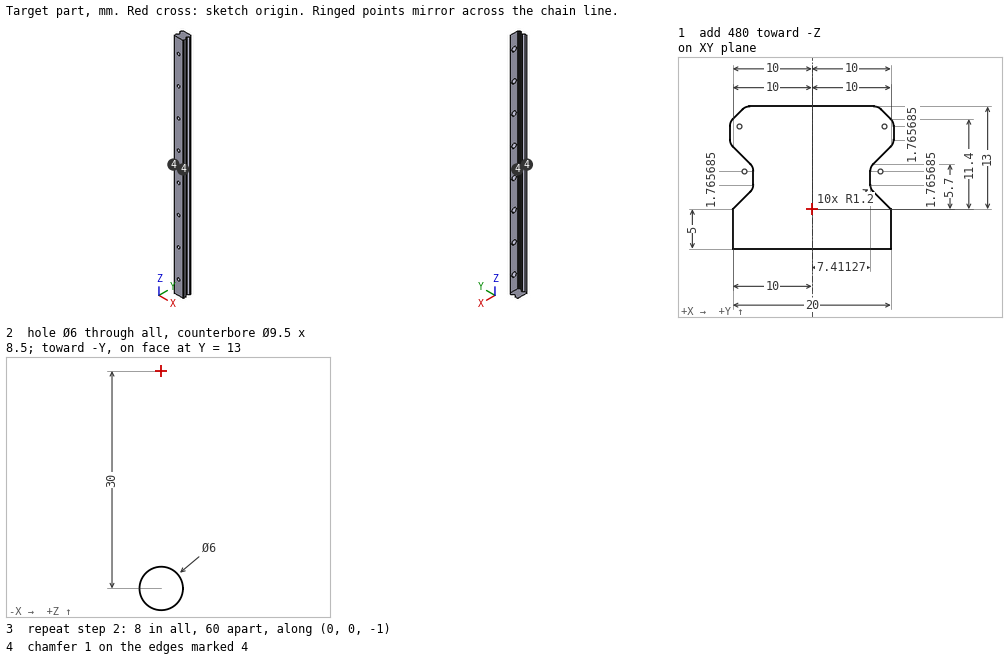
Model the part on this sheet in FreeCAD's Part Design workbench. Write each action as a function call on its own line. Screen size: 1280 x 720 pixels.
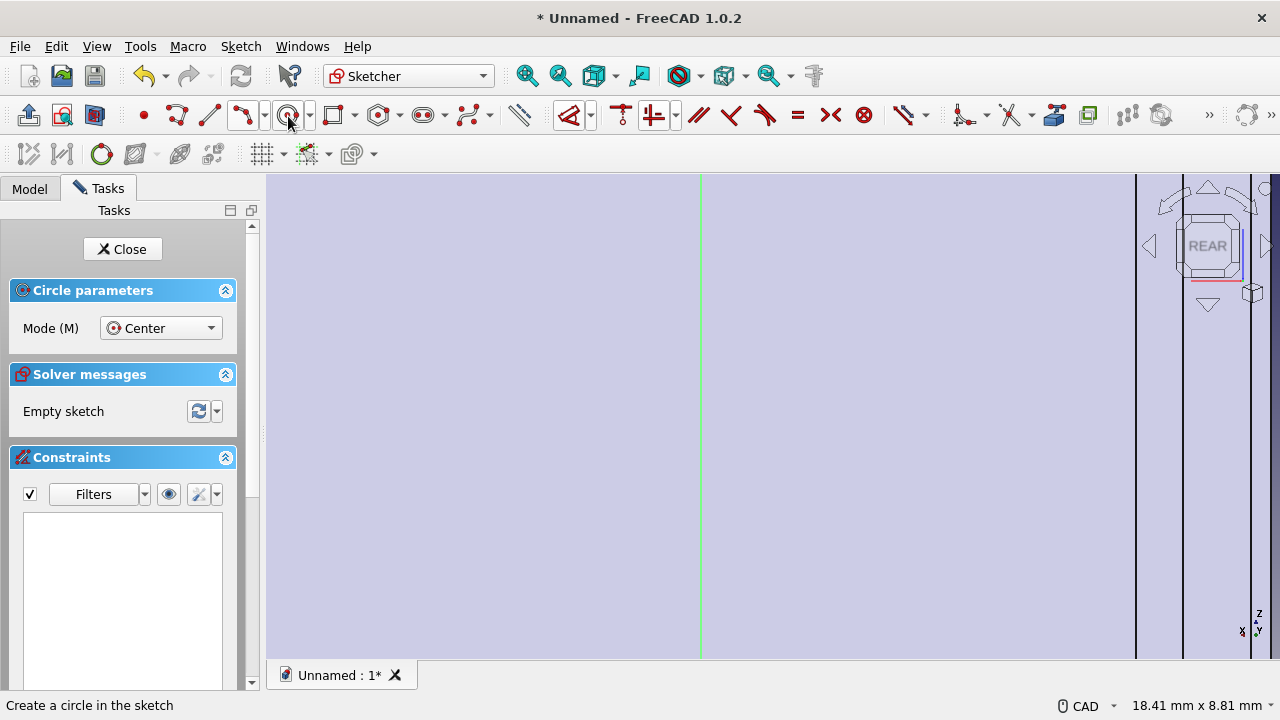
click(701, 413)
move(817, 296)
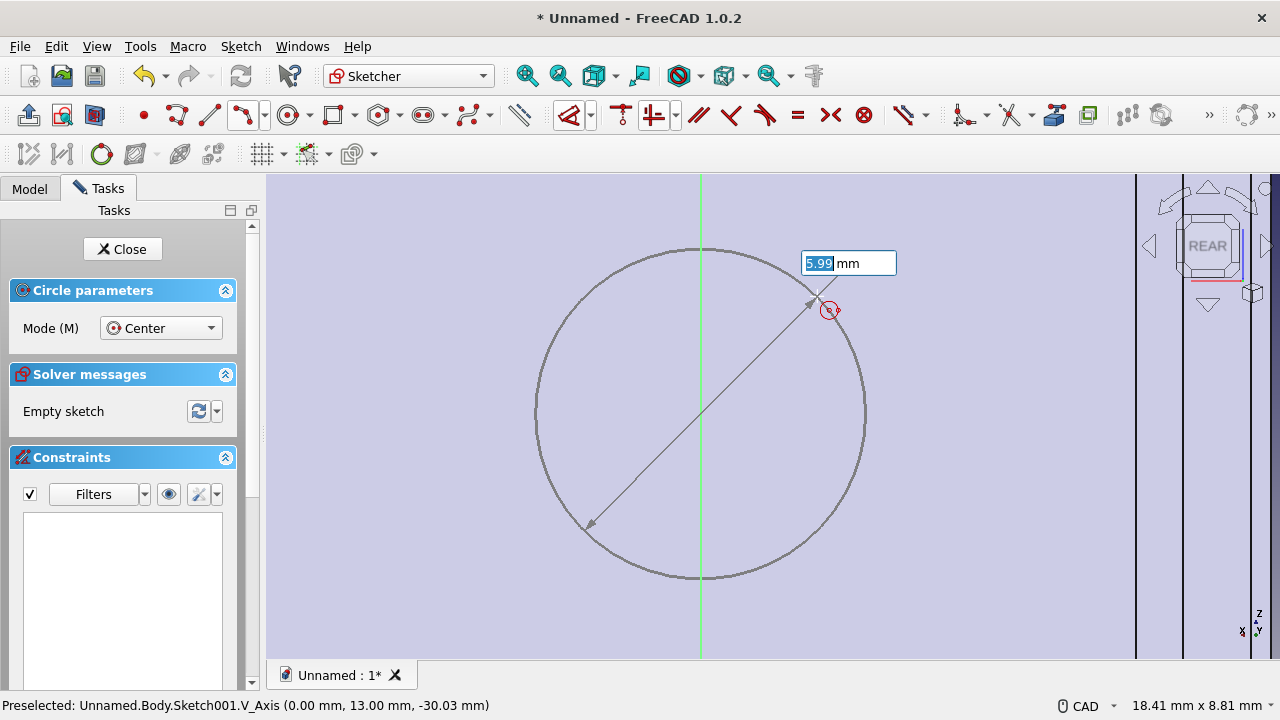
text(6)
key(Return)
key(Escape)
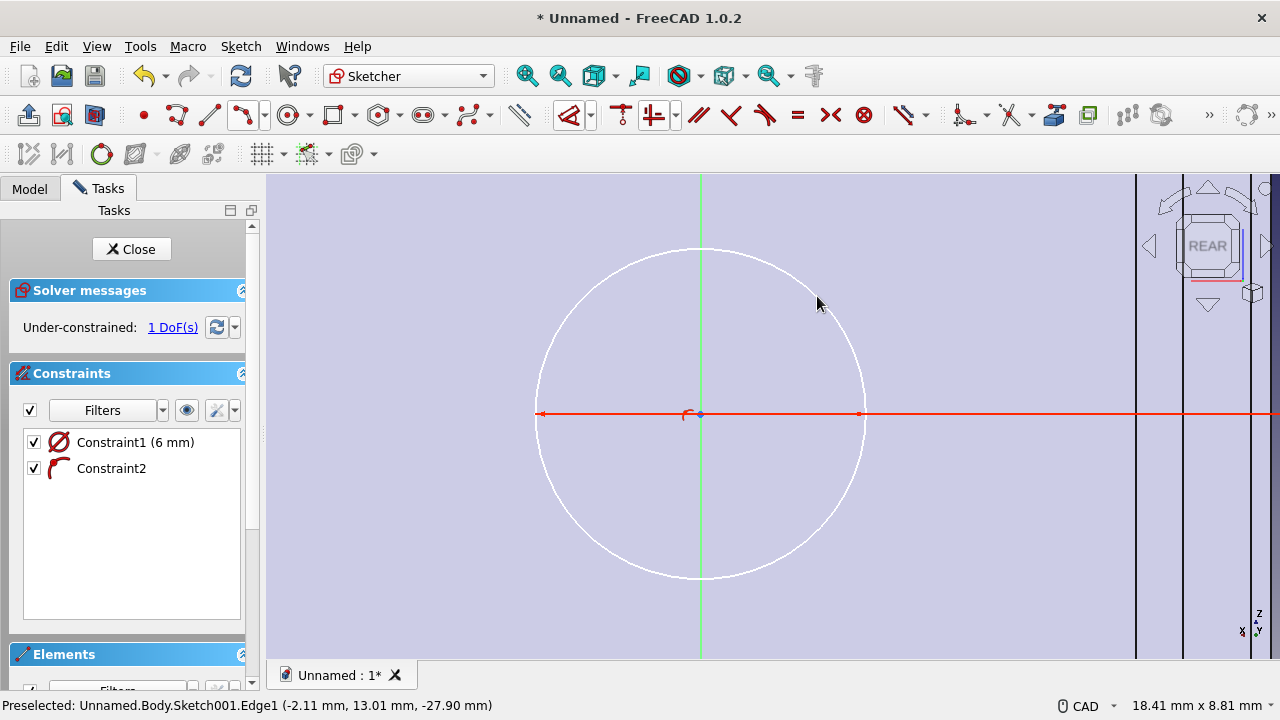
click(568, 116)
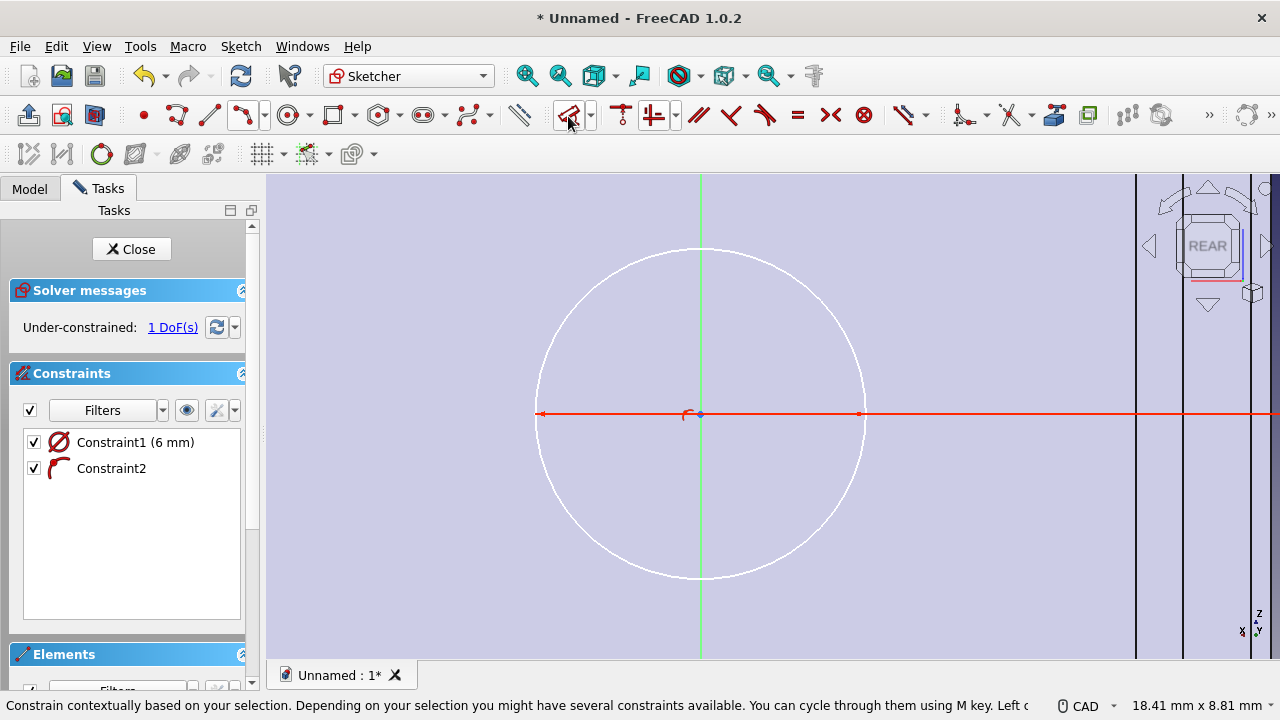
click(701, 414)
click(735, 308)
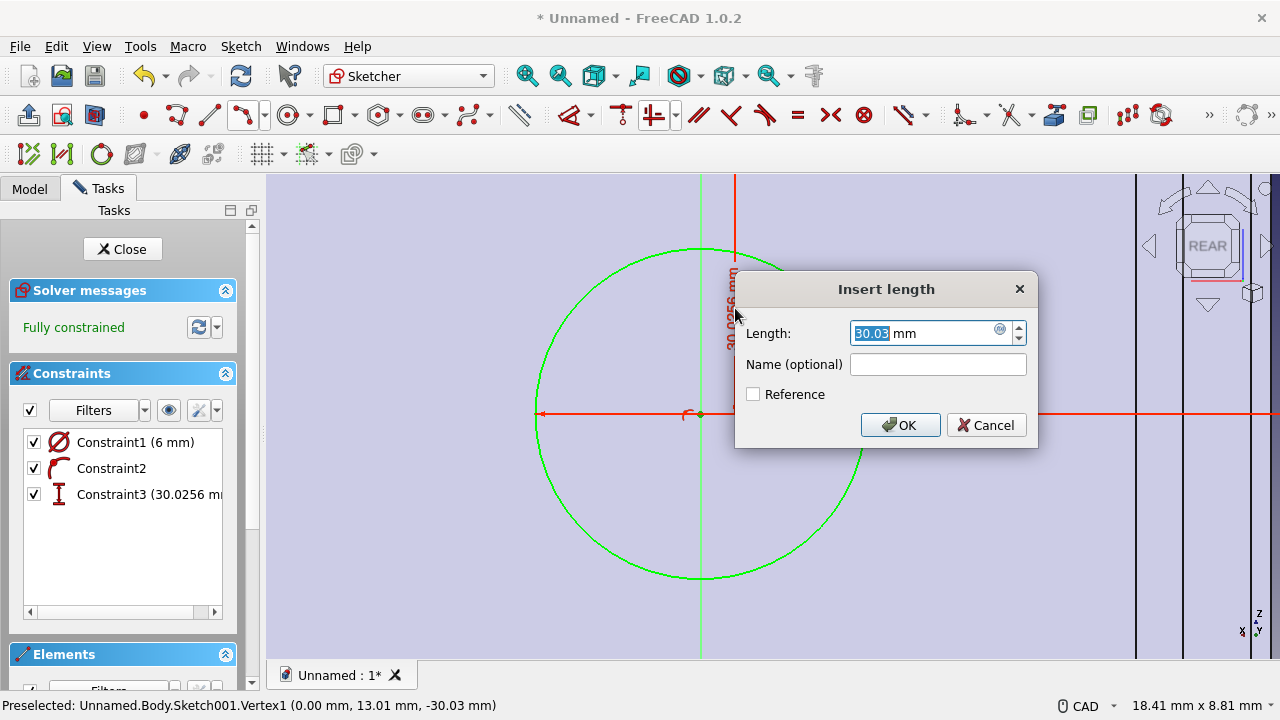
text(30)
key(Return)
key(Escape)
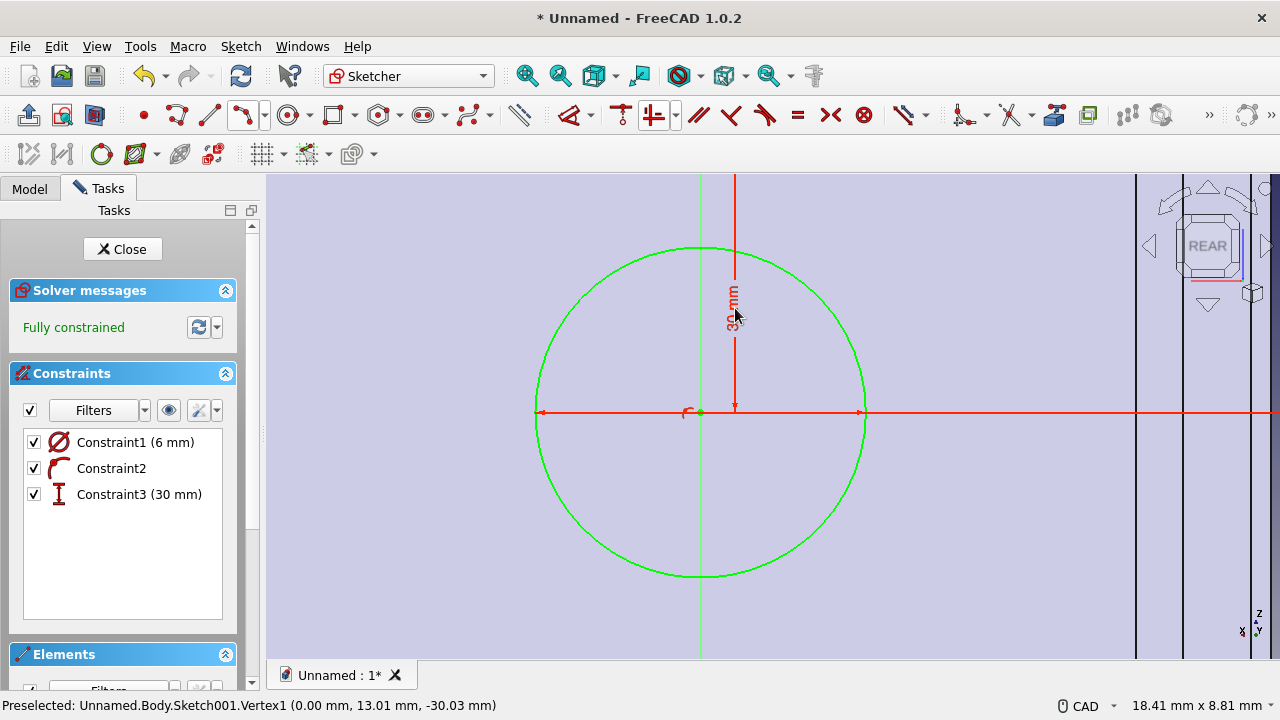
click(123, 249)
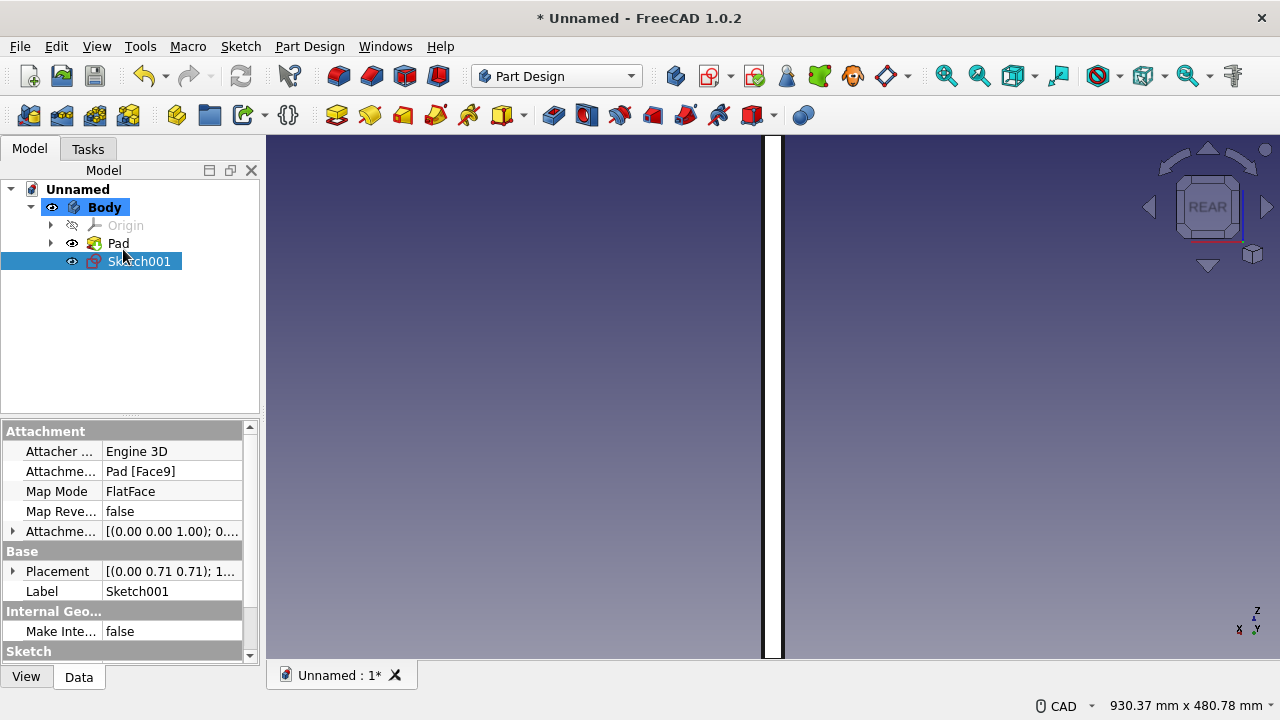
click(587, 116)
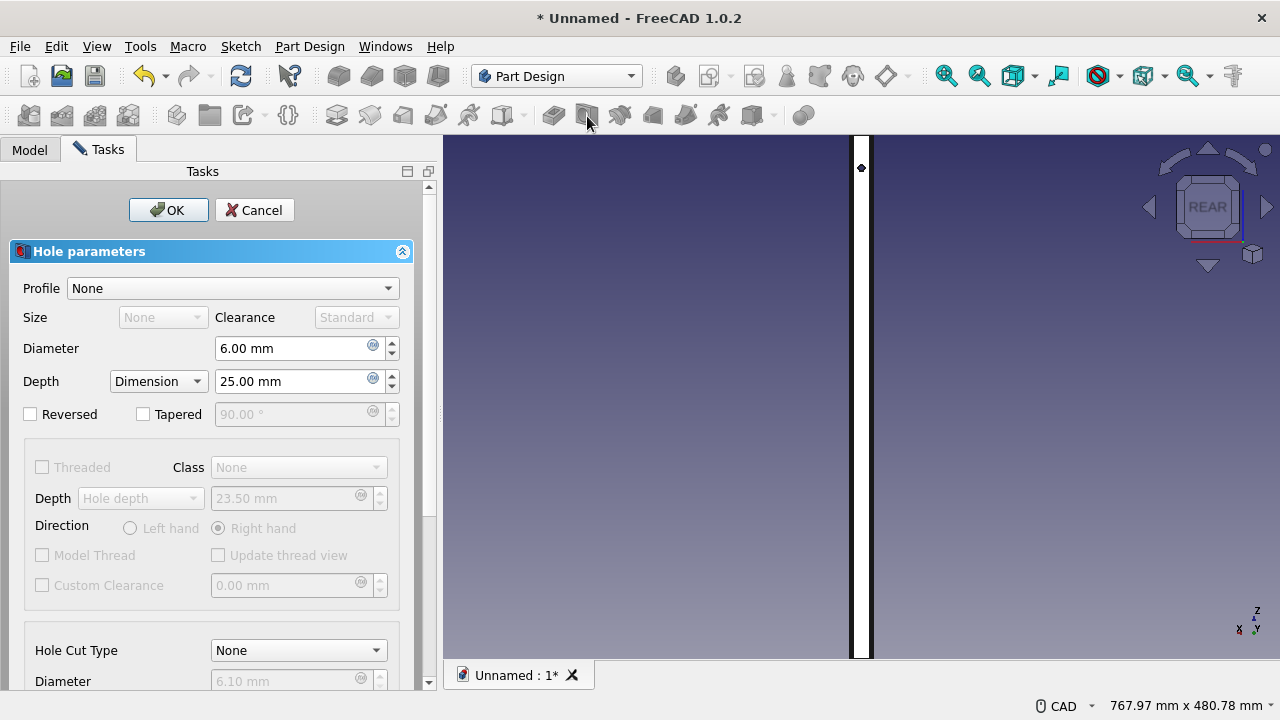
triple_click(300, 348)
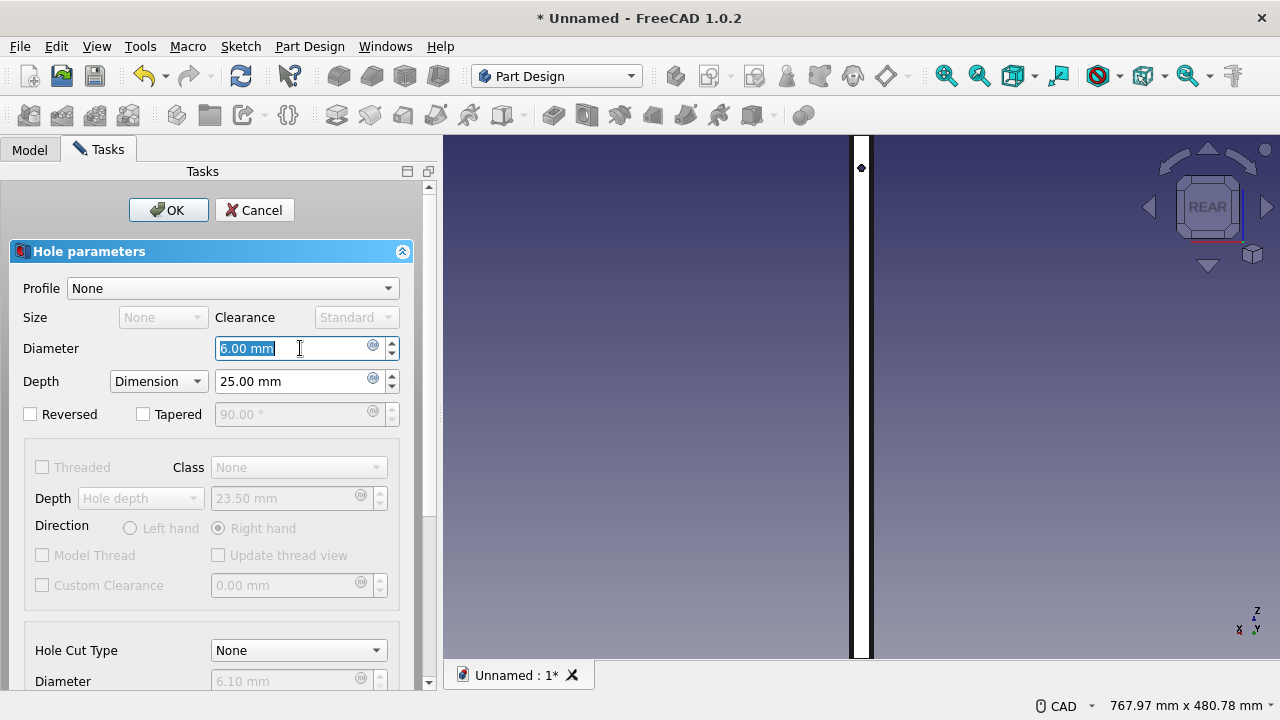
text(6)
key(Tab)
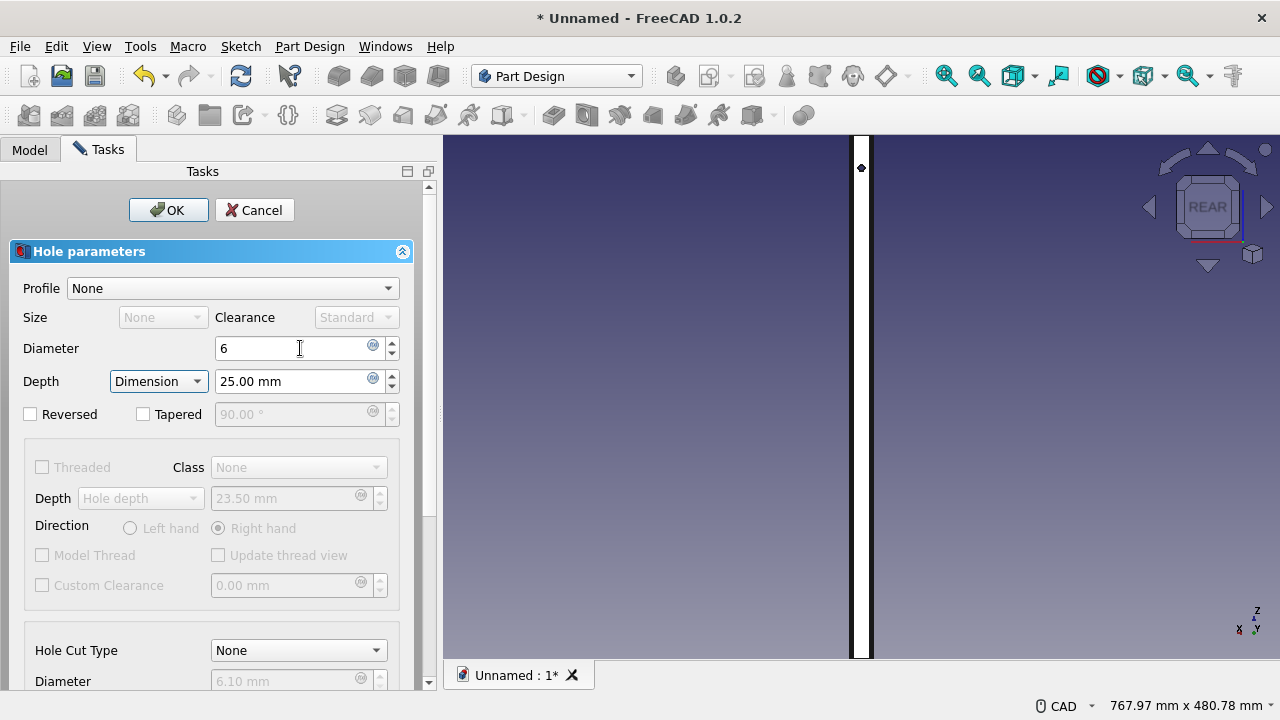
click(160, 382)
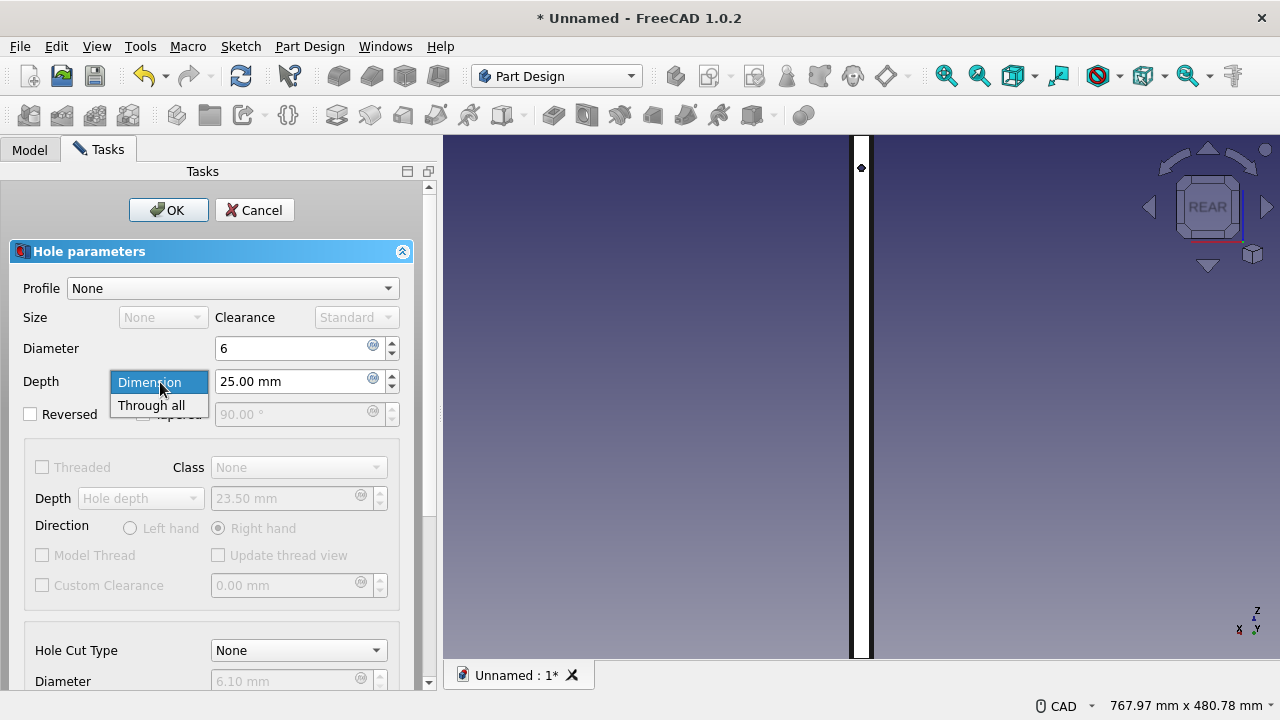
click(158, 406)